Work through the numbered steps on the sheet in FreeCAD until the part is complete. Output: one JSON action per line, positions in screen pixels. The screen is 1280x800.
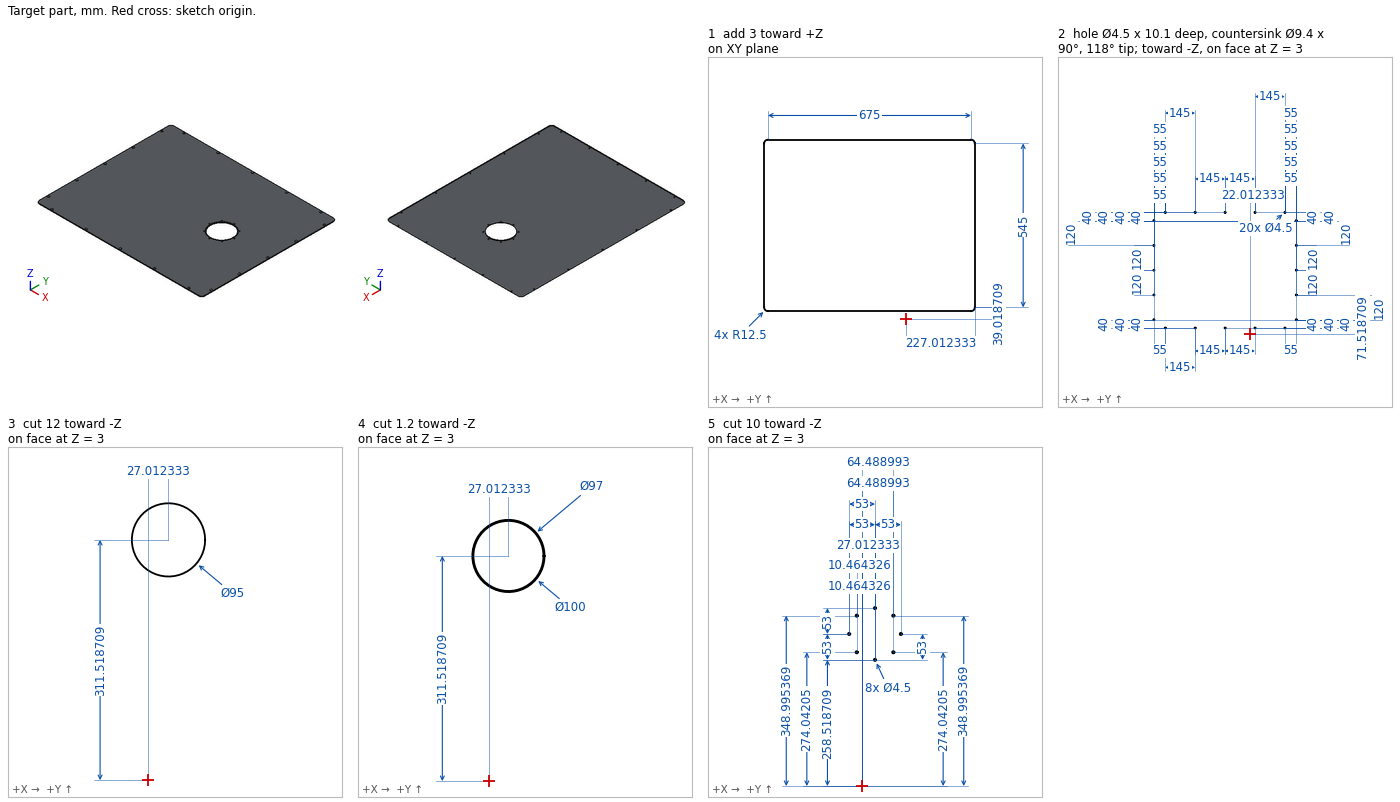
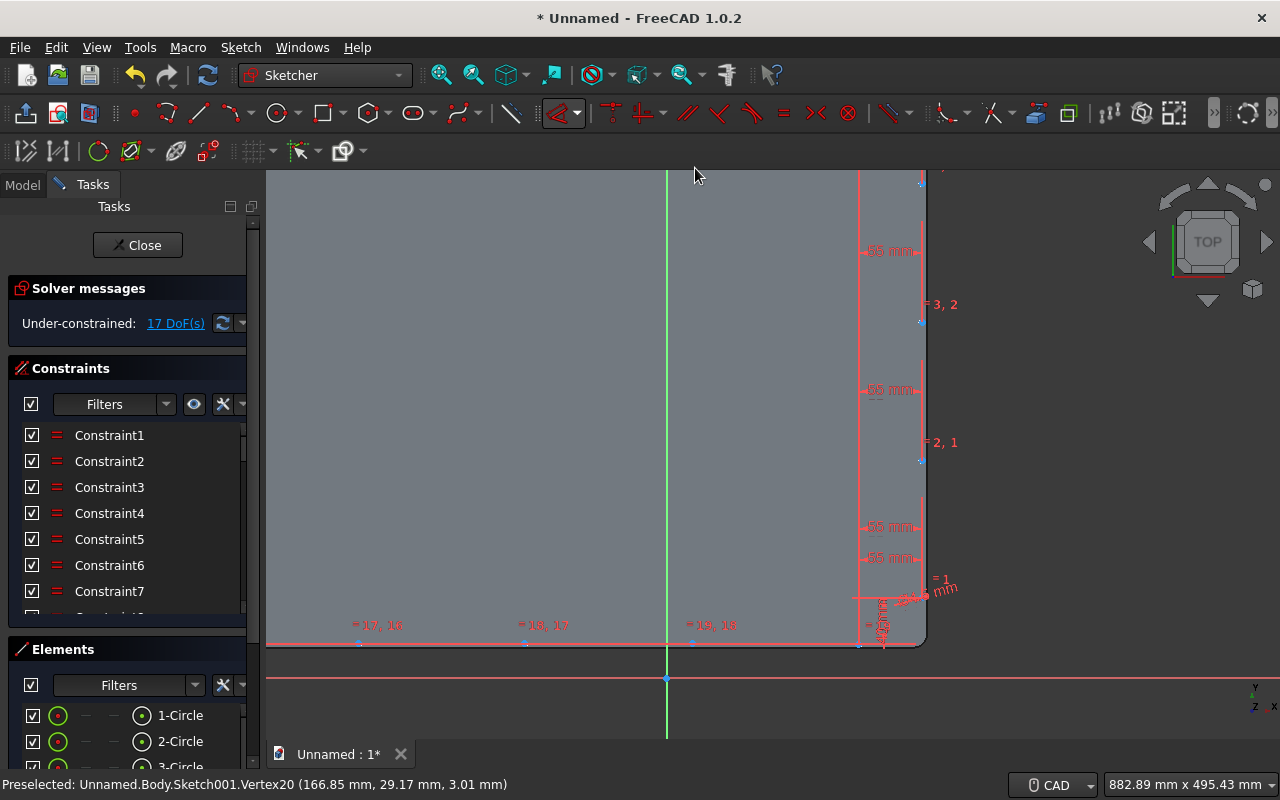
{"action": "left_click", "coordinate": [922, 598]}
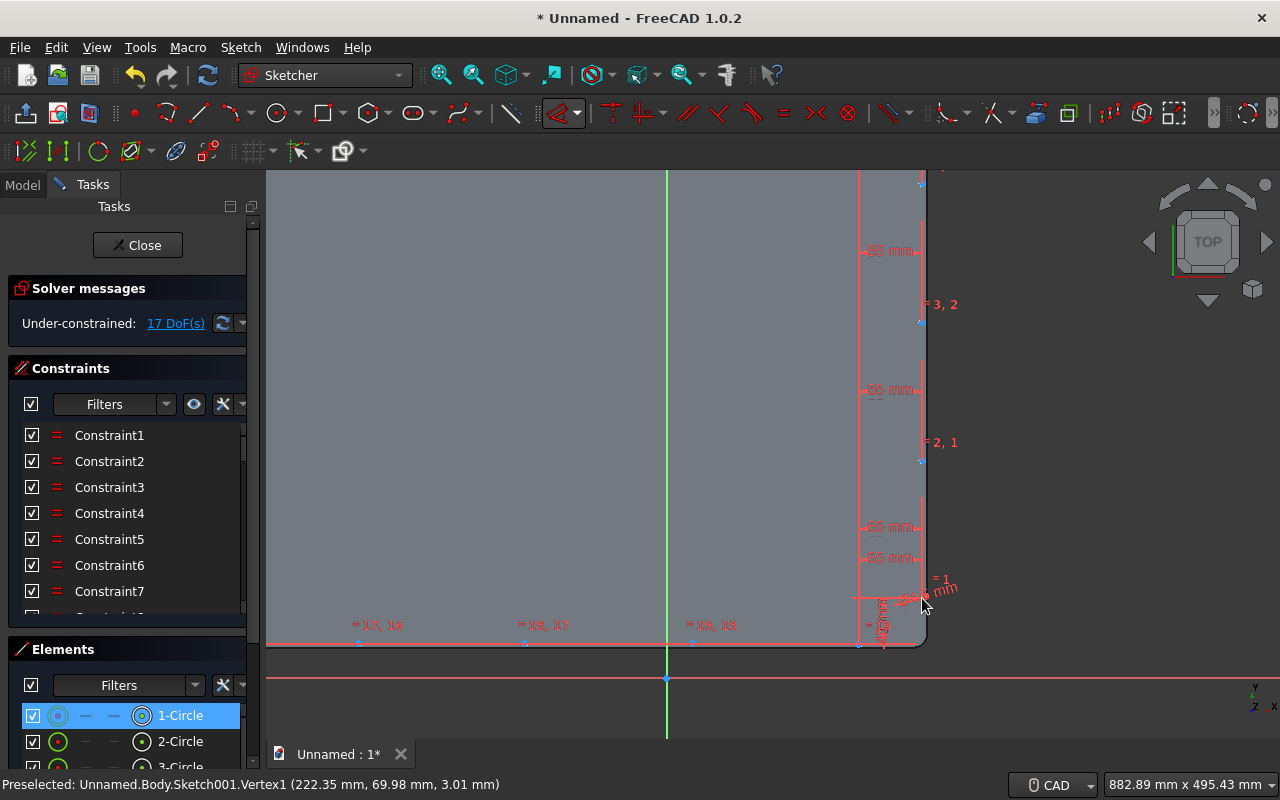
{"action": "left_click", "coordinate": [859, 645]}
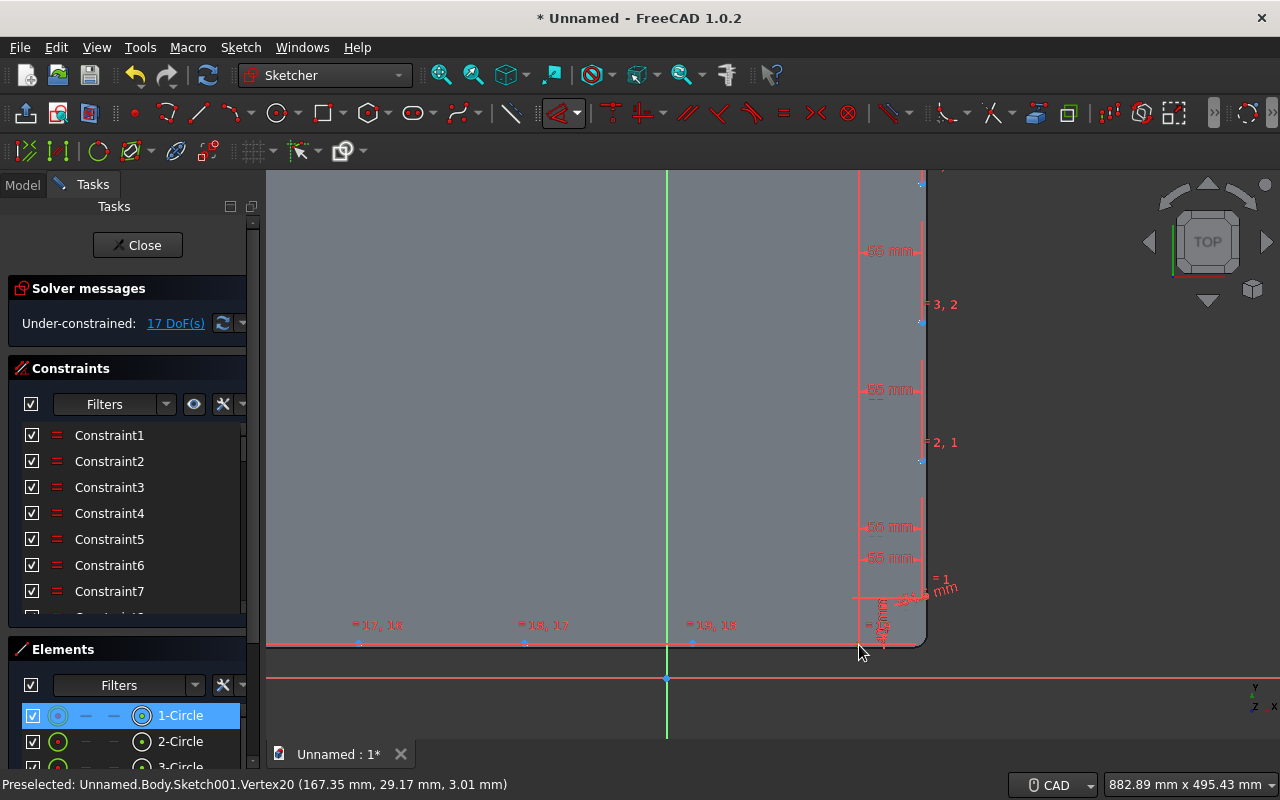
{"action": "left_click", "coordinate": [580, 114]}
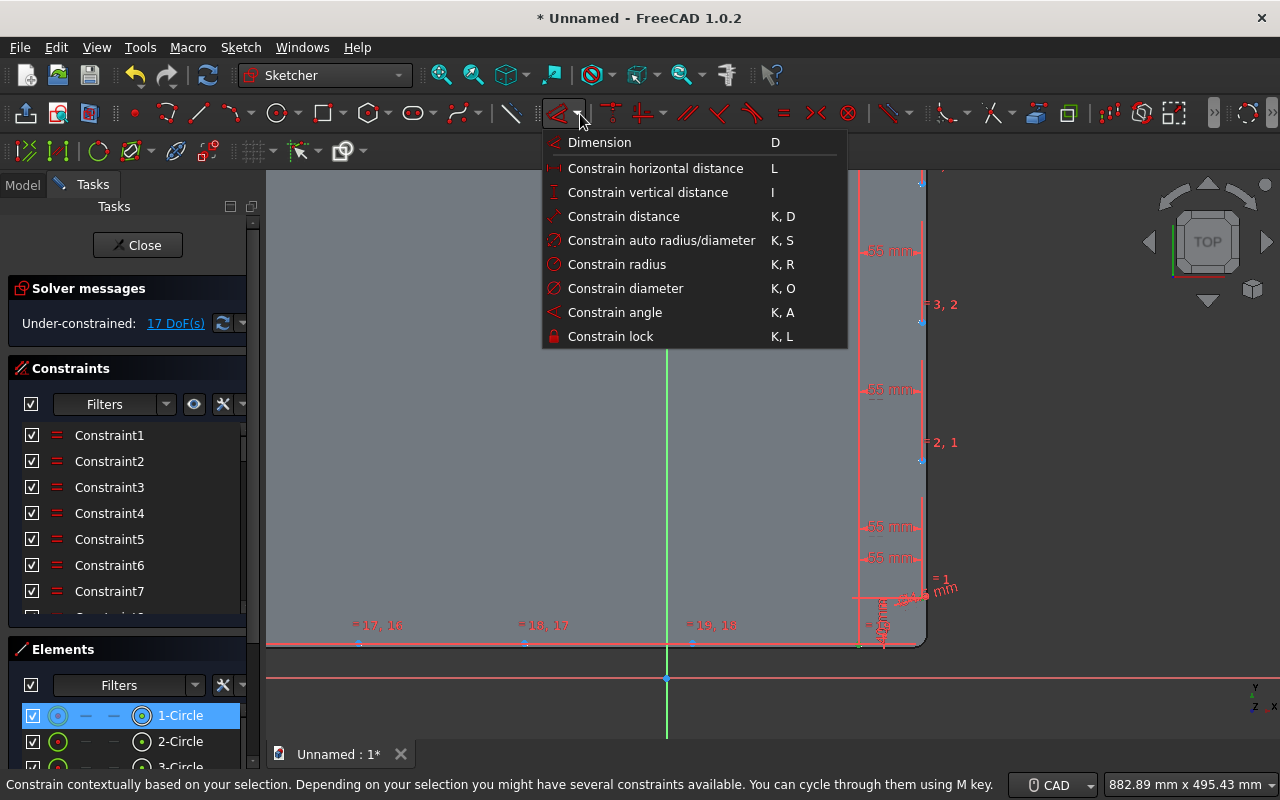
{"action": "left_click", "coordinate": [695, 192]}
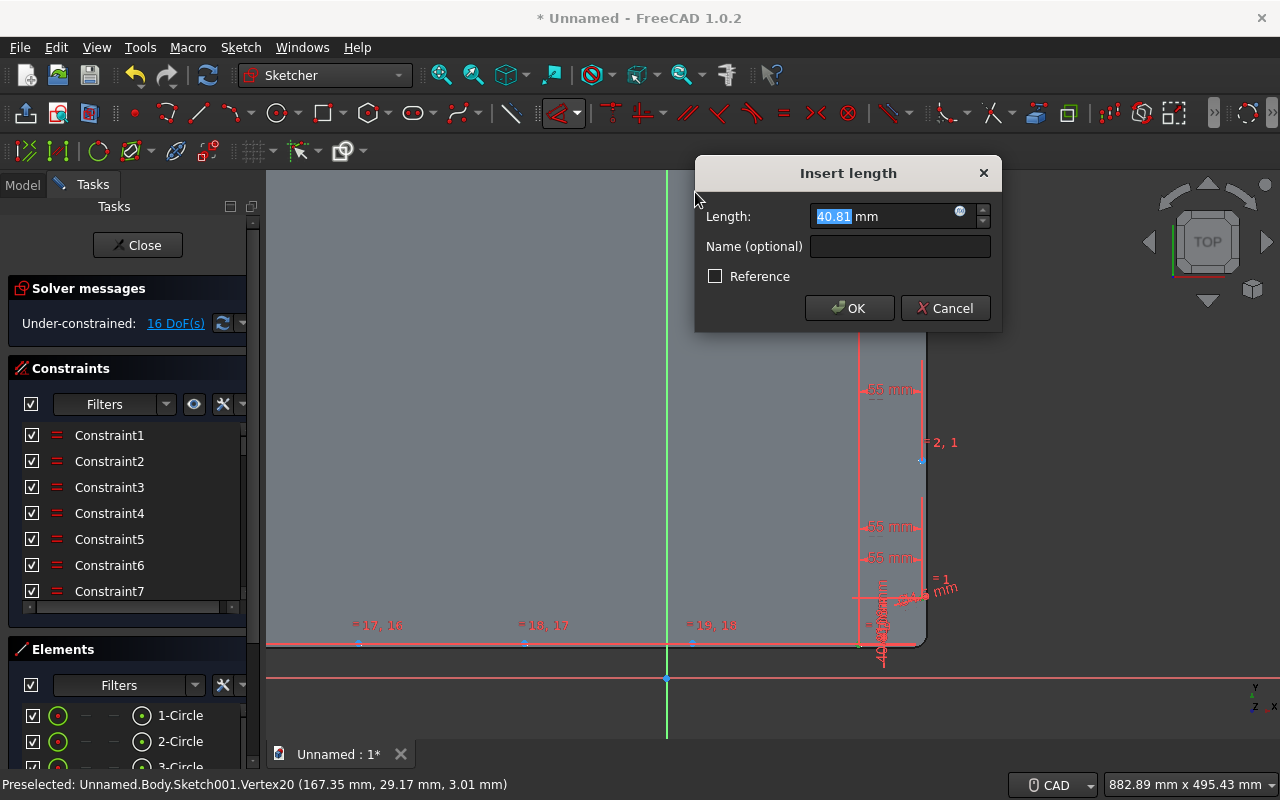
{"action": "type", "text": "40"}
{"action": "key", "text": "Return"}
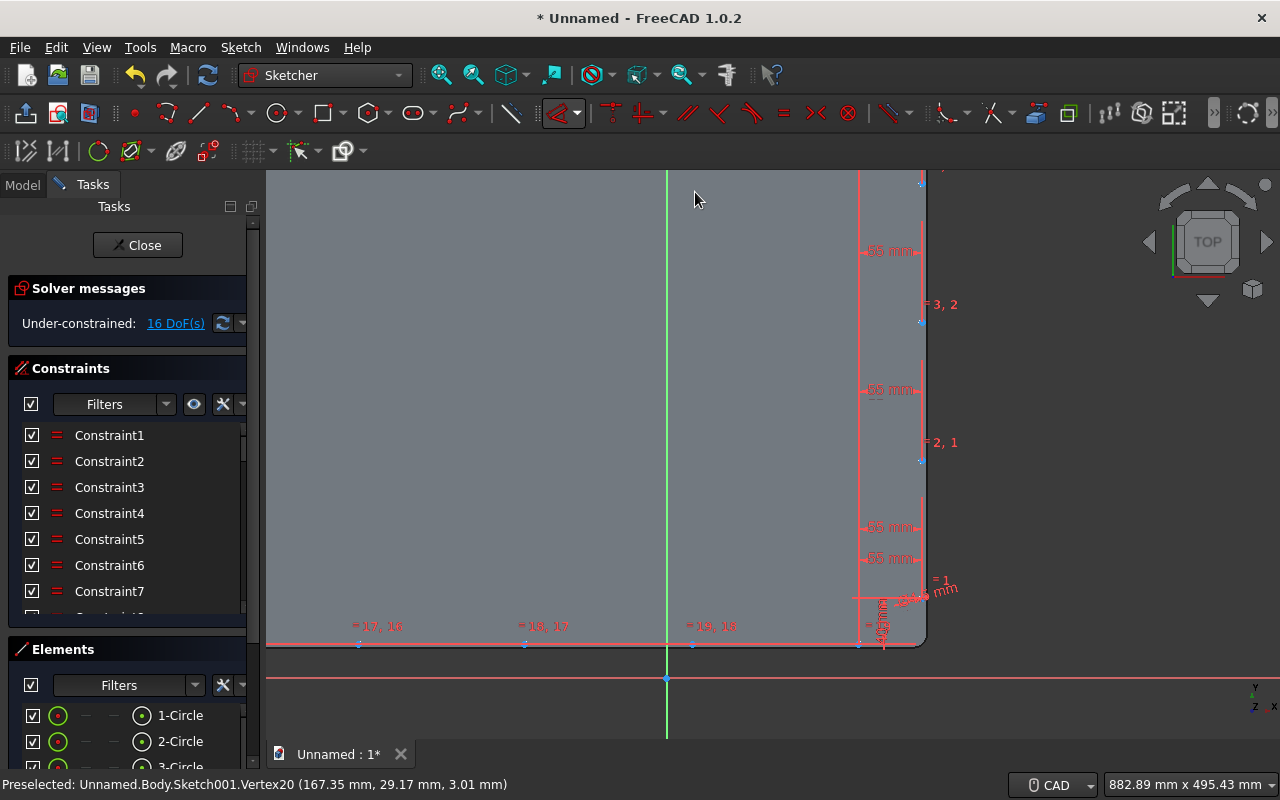
{"action": "left_click", "coordinate": [922, 598]}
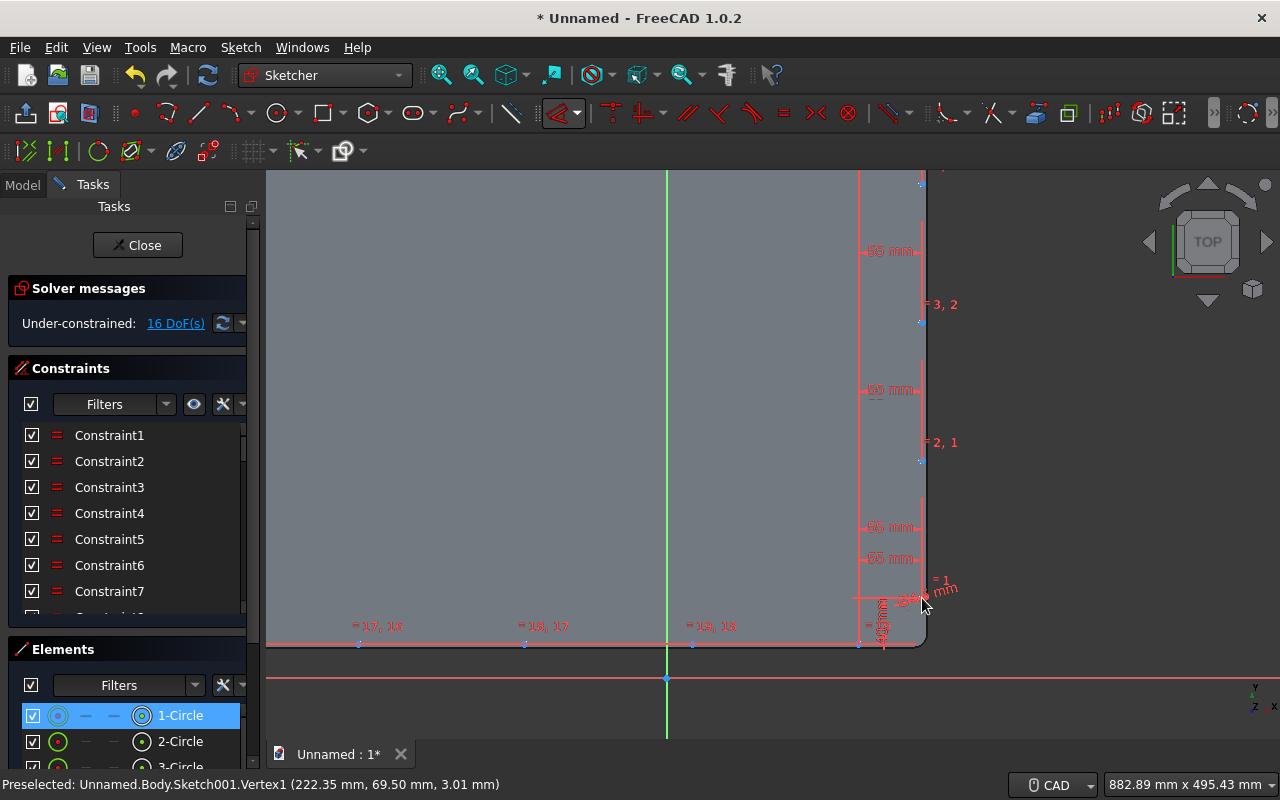
{"action": "left_click", "coordinate": [922, 461]}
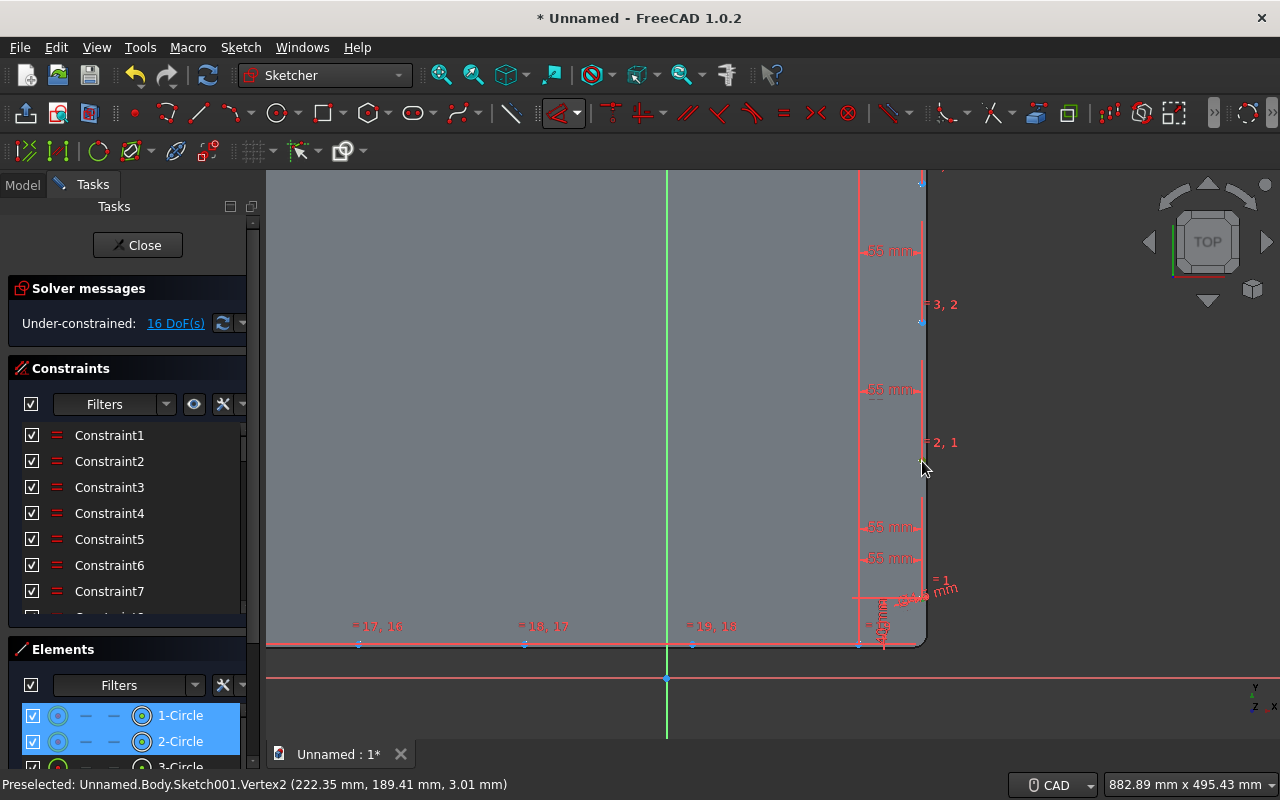
{"action": "left_click", "coordinate": [580, 114]}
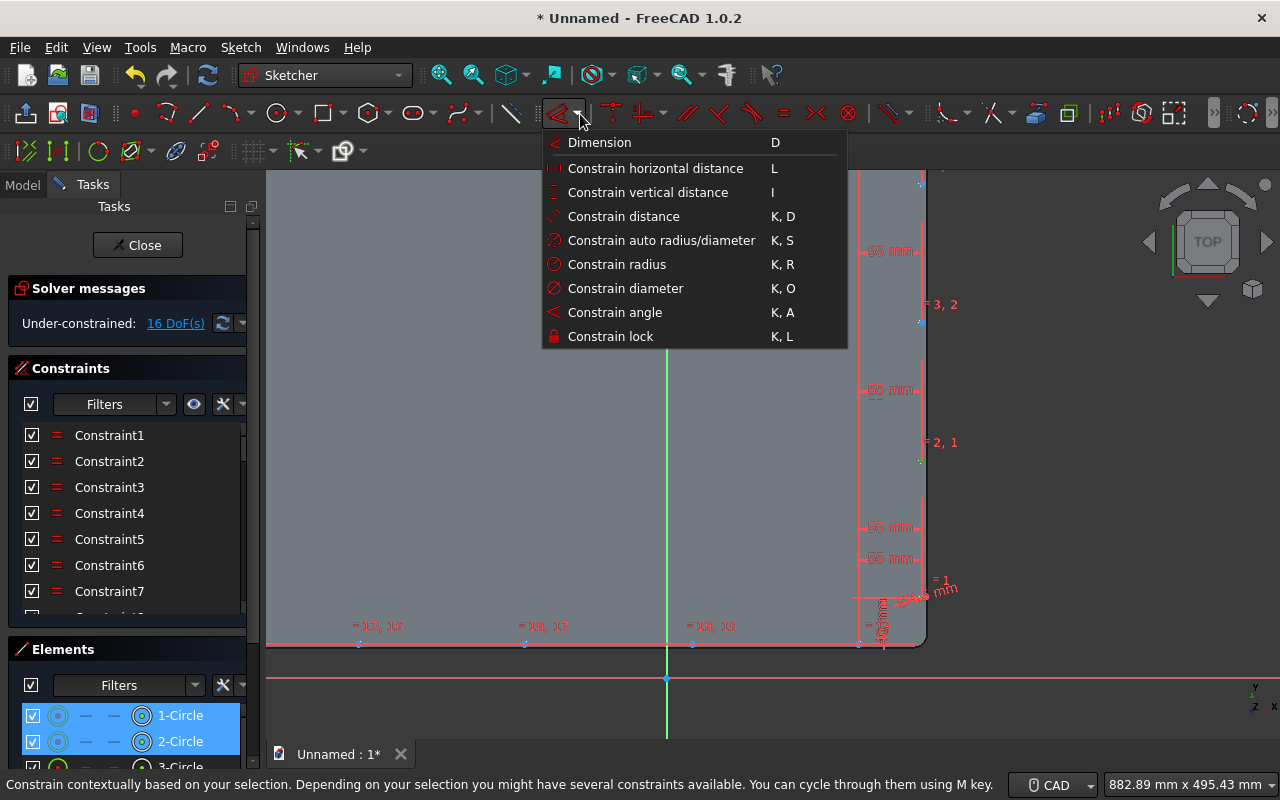
{"action": "left_click", "coordinate": [695, 192]}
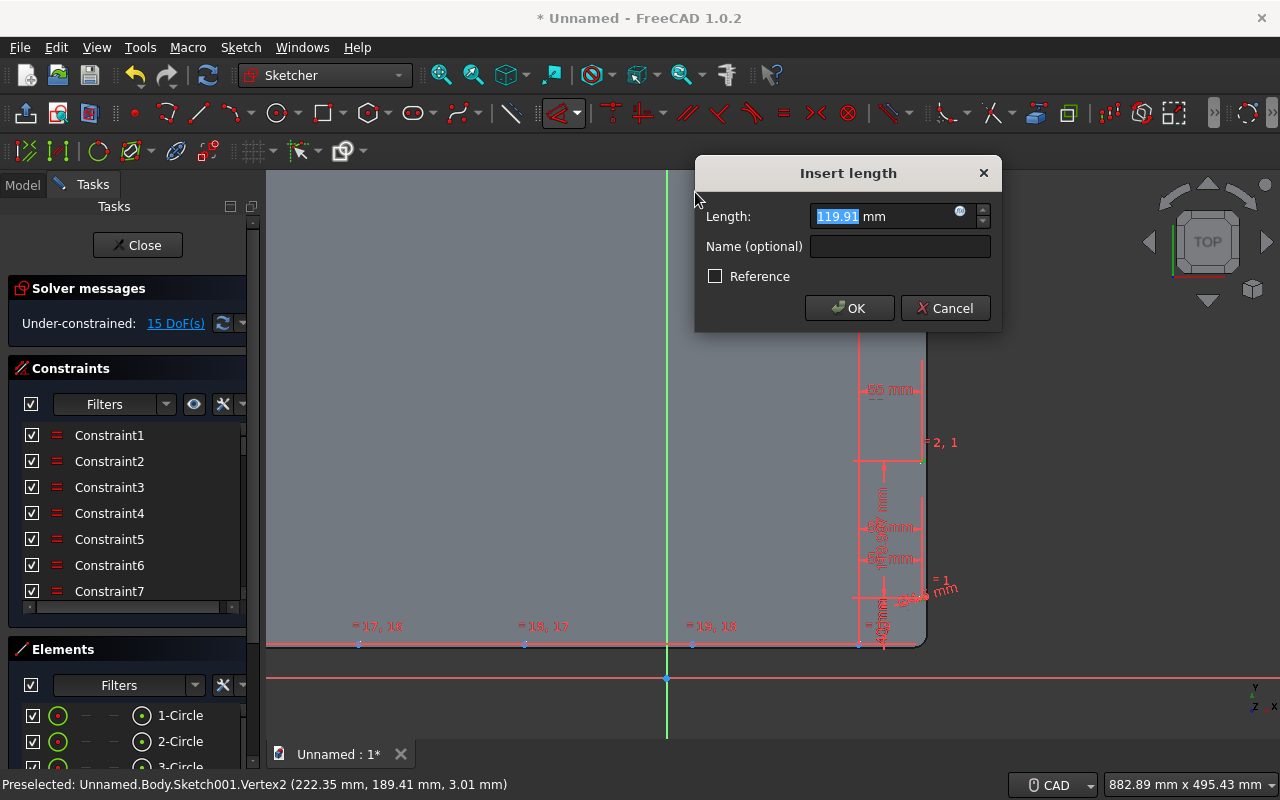
{"action": "type", "text": "120"}
{"action": "key", "text": "Return"}